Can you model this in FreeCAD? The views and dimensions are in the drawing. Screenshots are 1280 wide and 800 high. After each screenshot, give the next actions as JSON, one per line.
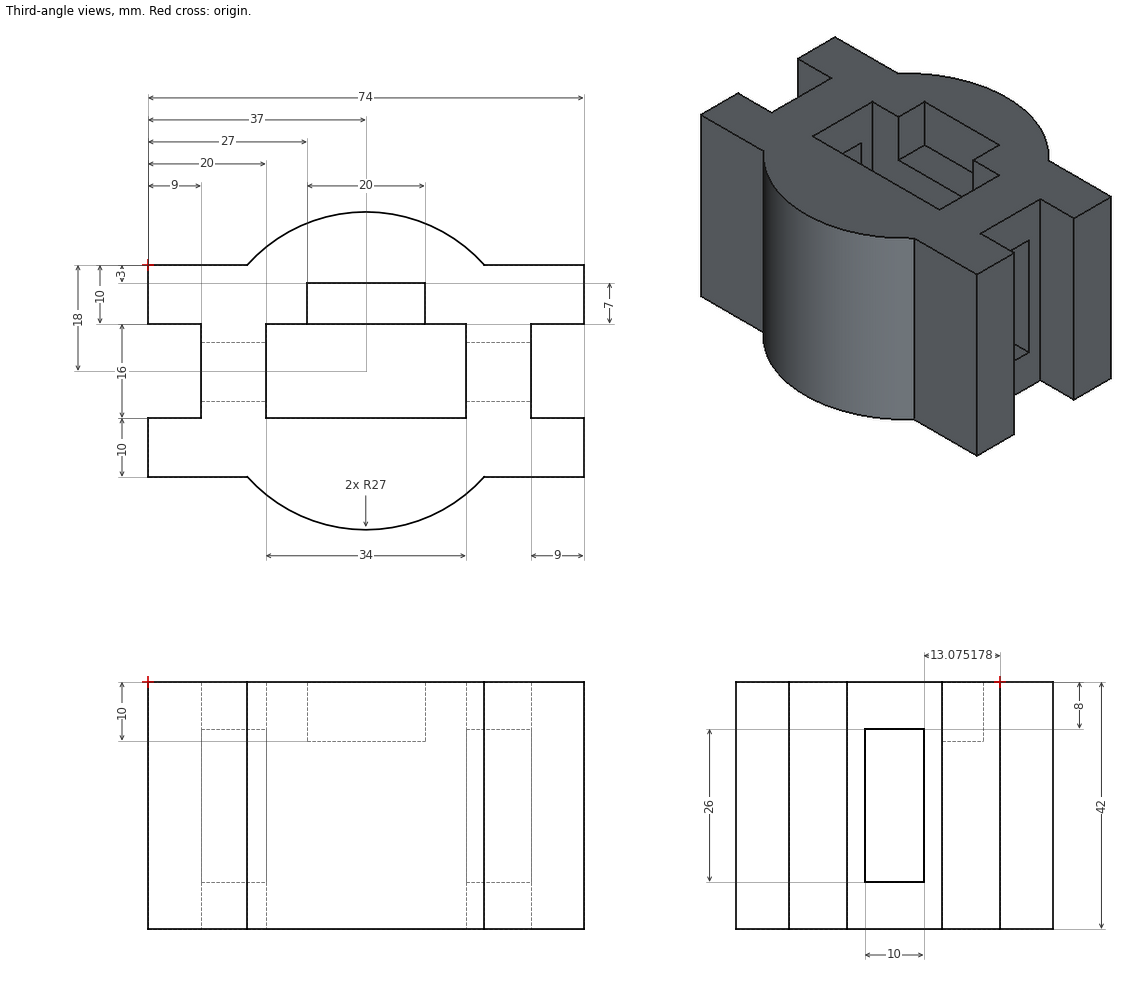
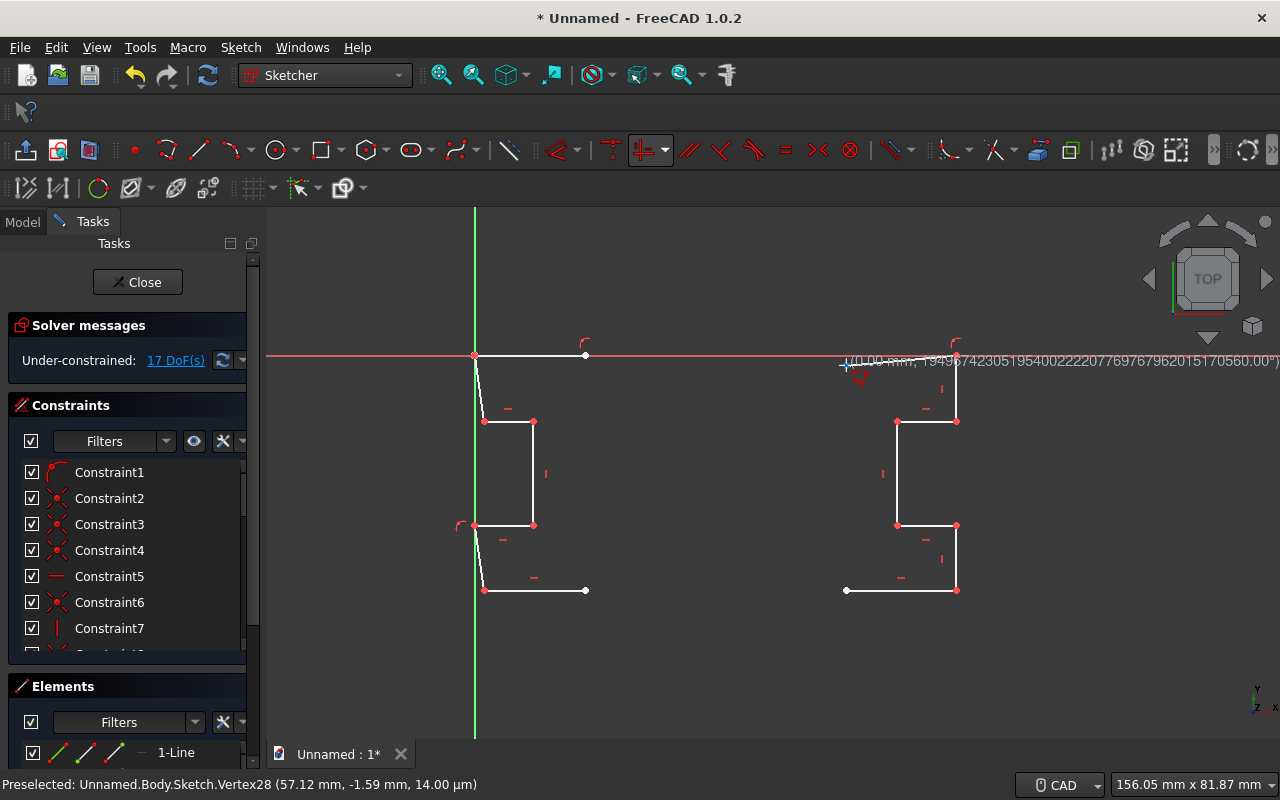
{"action": "left_click", "coordinate": [232, 150]}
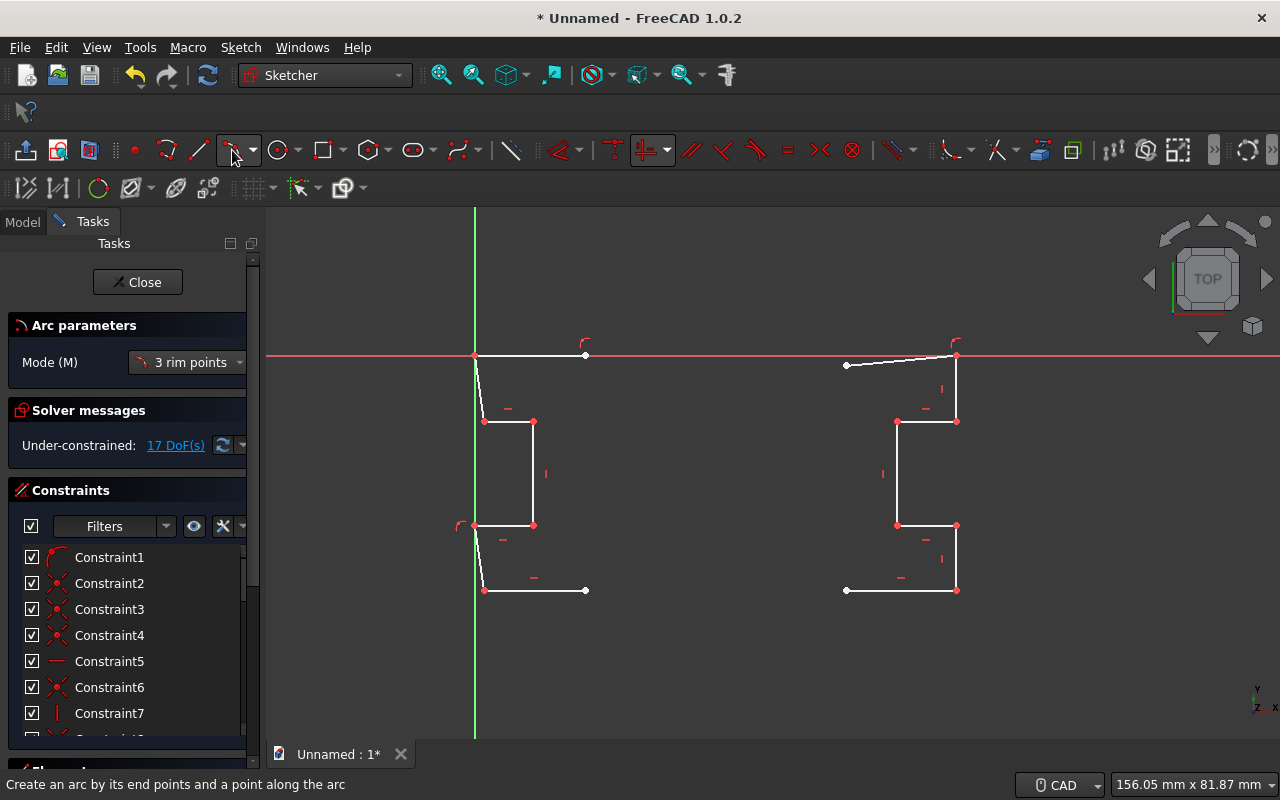
{"action": "left_click", "coordinate": [585, 591]}
{"action": "left_click", "coordinate": [846, 591]}
{"action": "left_click", "coordinate": [715, 648]}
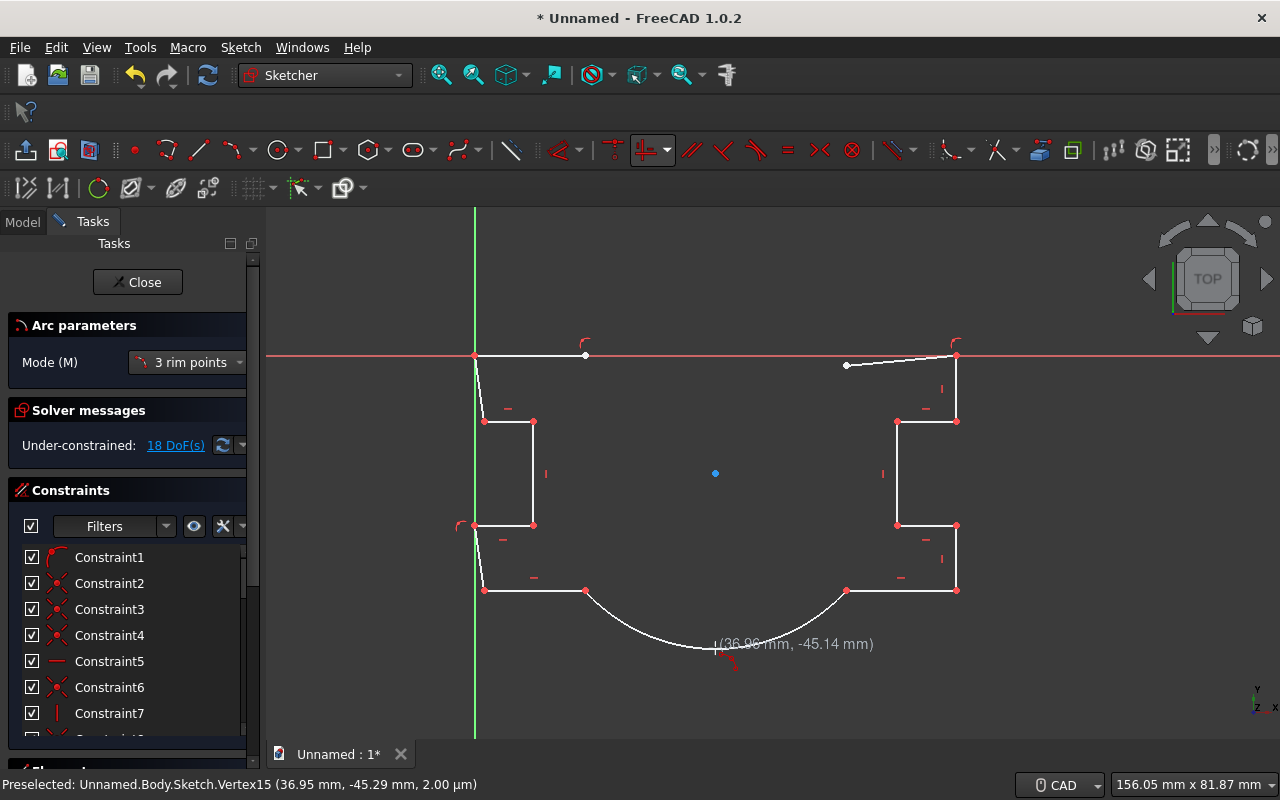
{"action": "left_click", "coordinate": [846, 366]}
{"action": "left_click", "coordinate": [585, 356]}
{"action": "left_click", "coordinate": [715, 297]}
{"action": "key", "text": "Escape"}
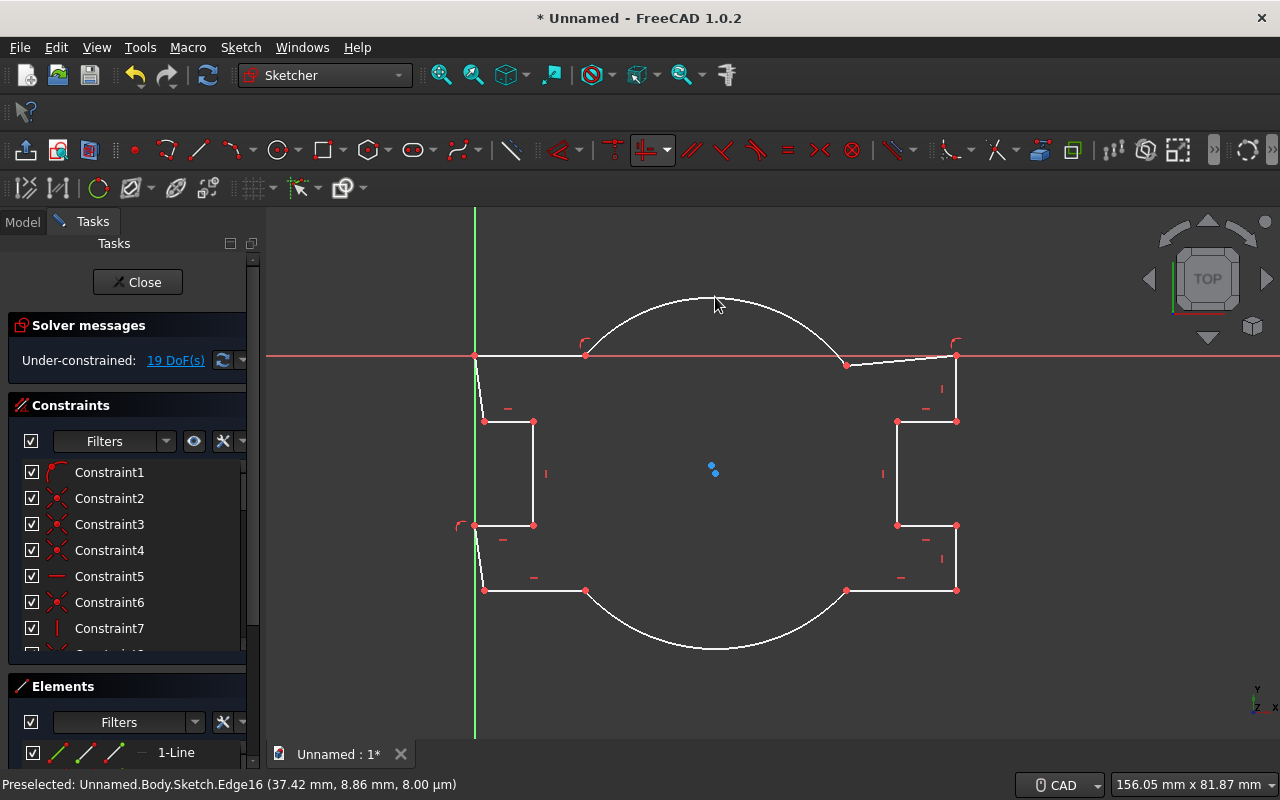
{"action": "left_click", "coordinate": [478, 376]}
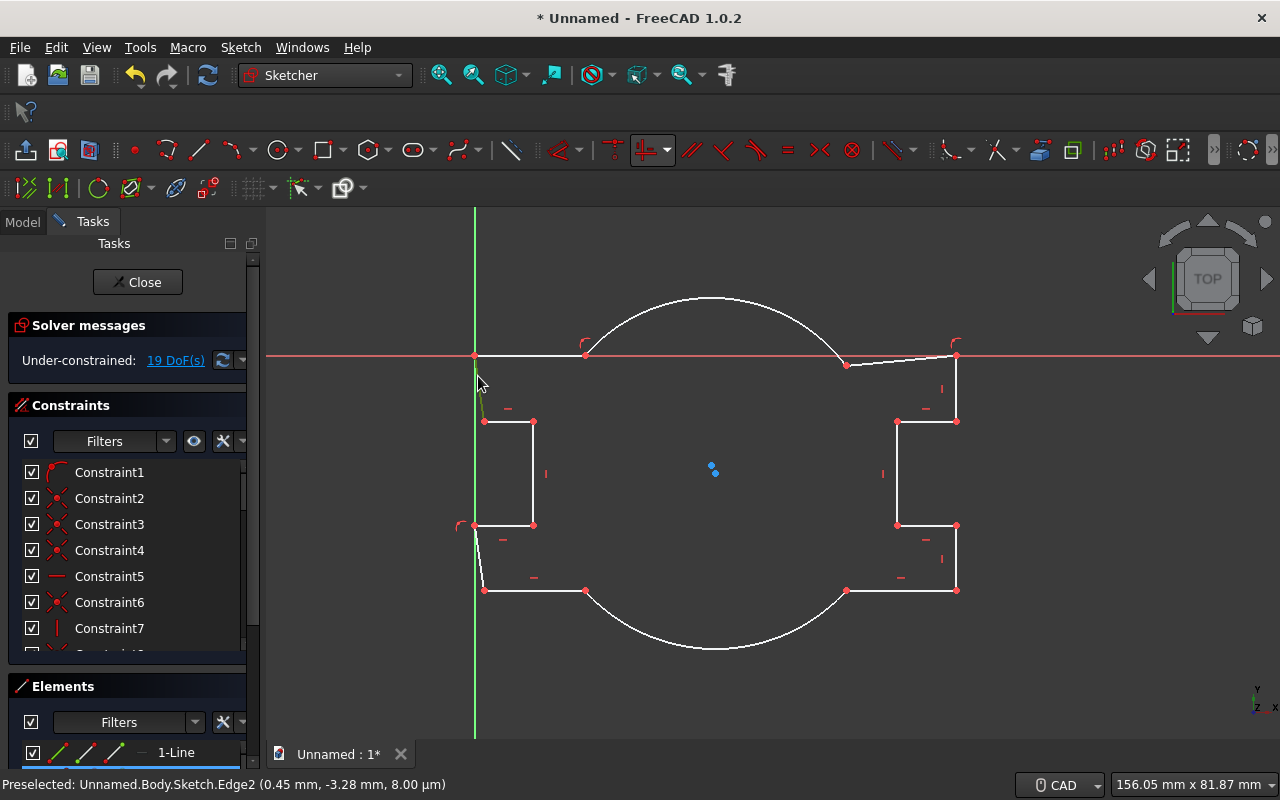
{"action": "key", "text": "v"}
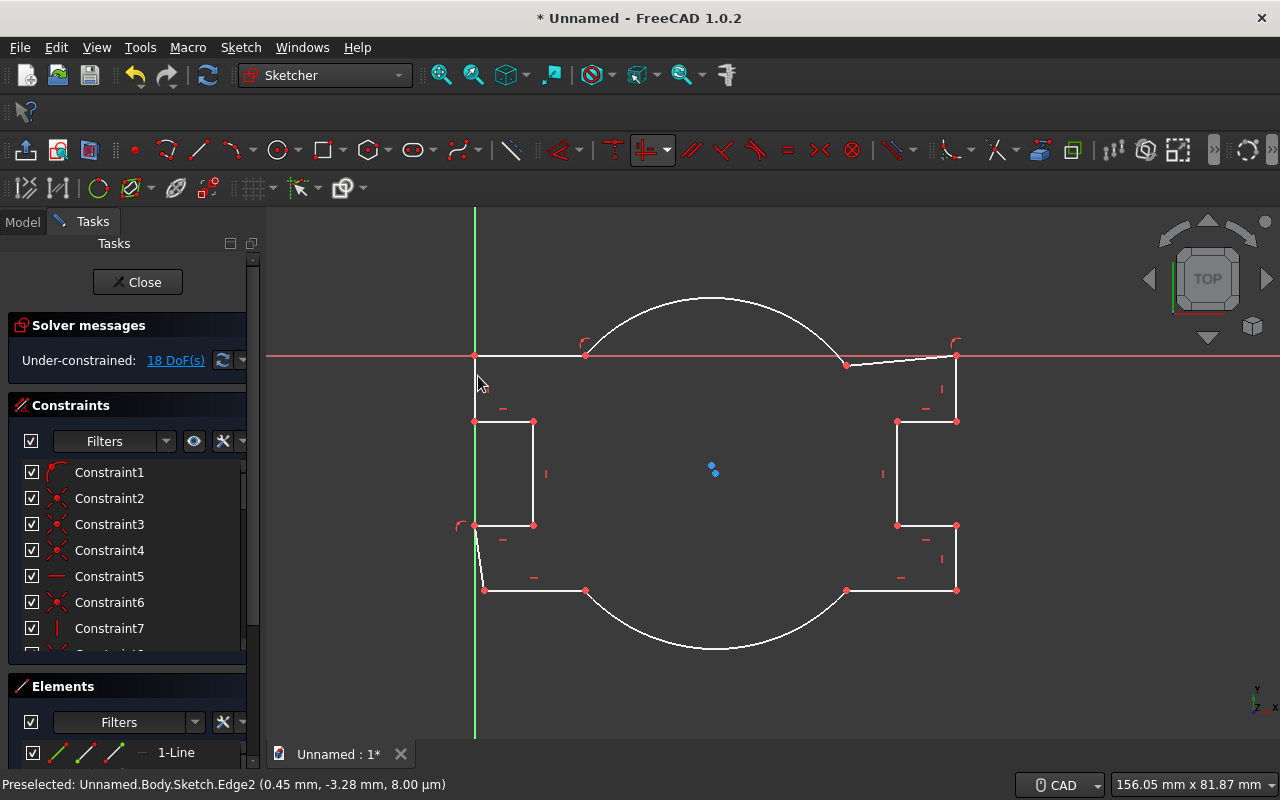
{"action": "left_click", "coordinate": [478, 546]}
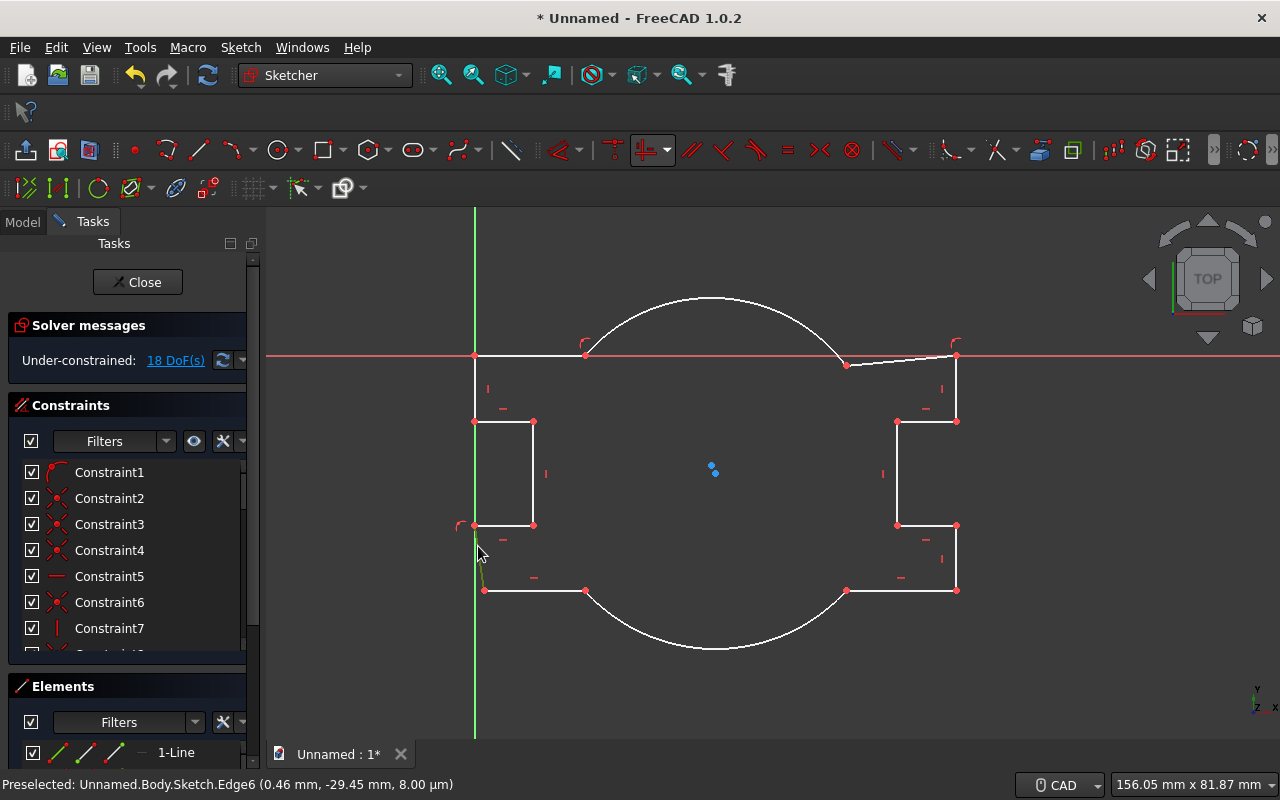
{"action": "left_click", "coordinate": [670, 150]}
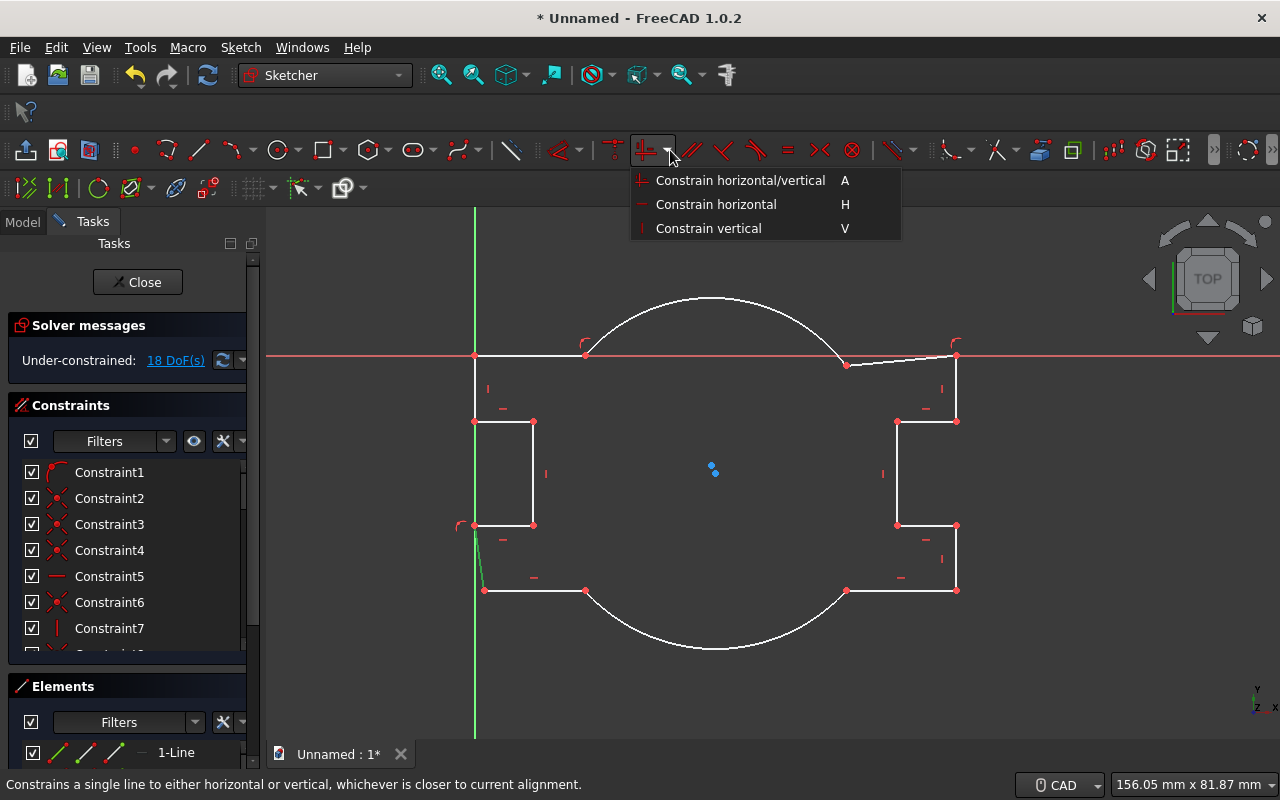
{"action": "left_click", "coordinate": [766, 228]}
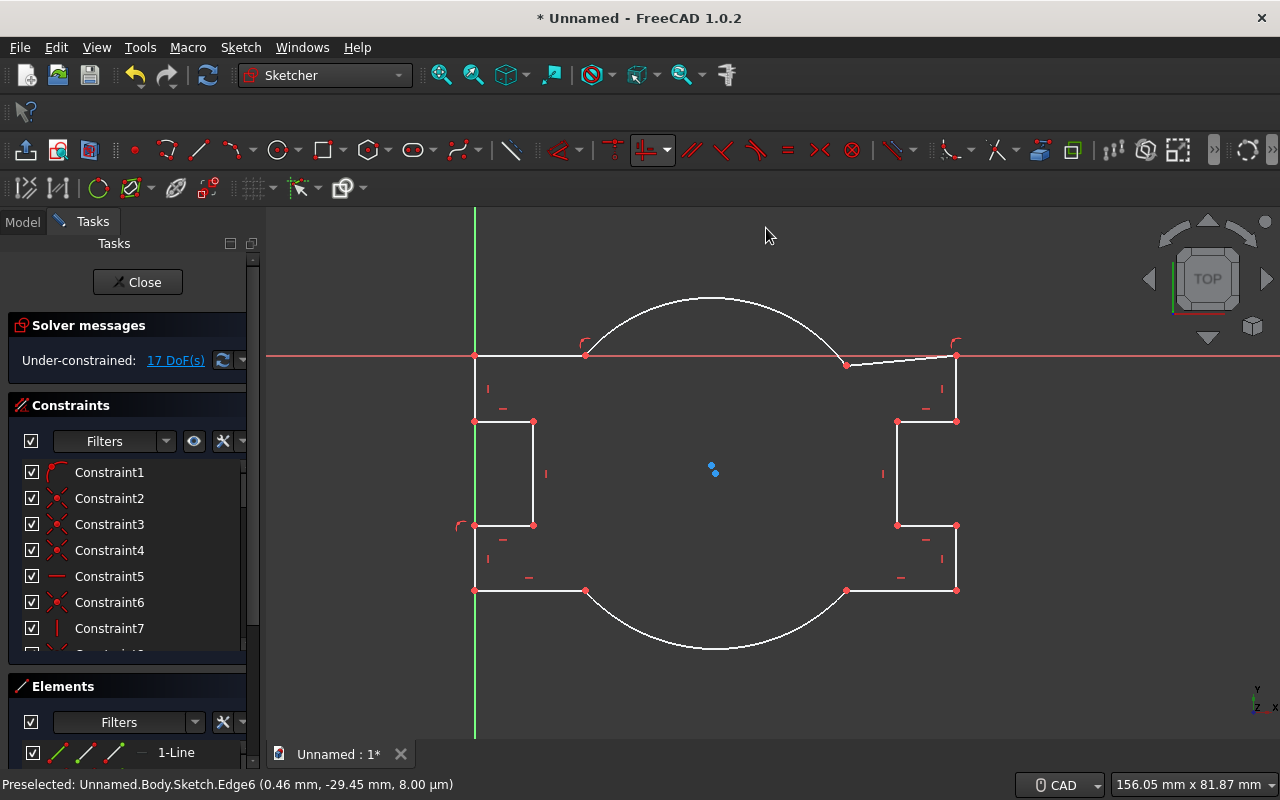
{"action": "left_click", "coordinate": [923, 359]}